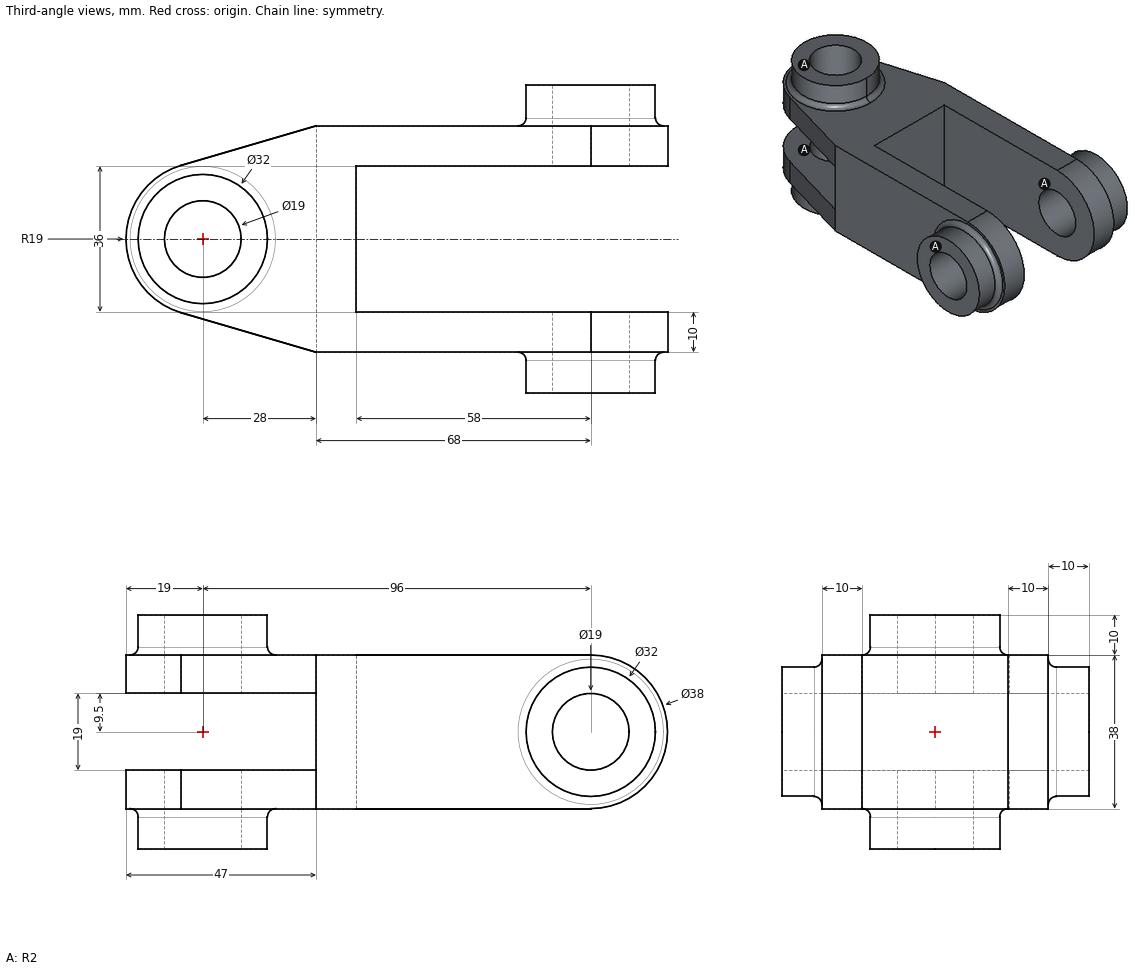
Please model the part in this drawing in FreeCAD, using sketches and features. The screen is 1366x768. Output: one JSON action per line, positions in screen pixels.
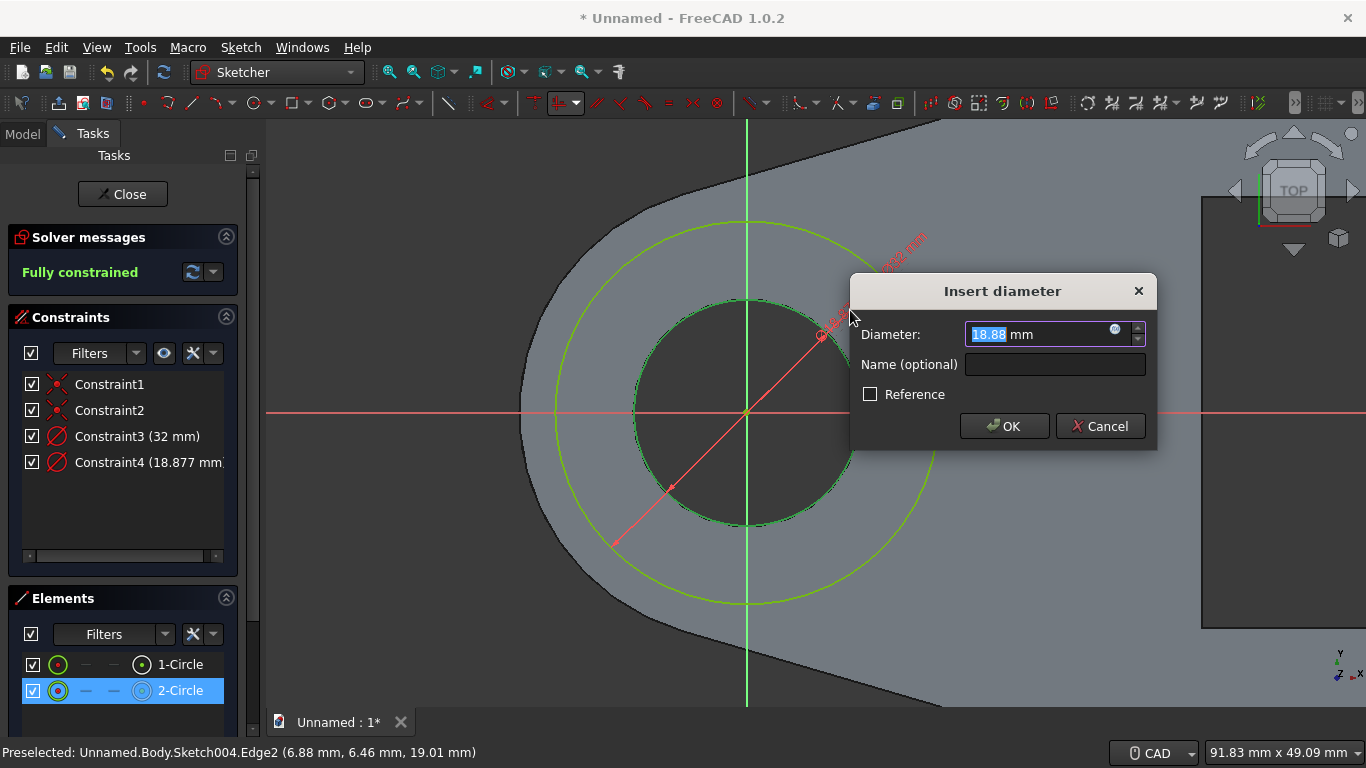
{"action": "type", "text": "19"}
{"action": "key", "text": "Return"}
{"action": "key", "text": "Escape"}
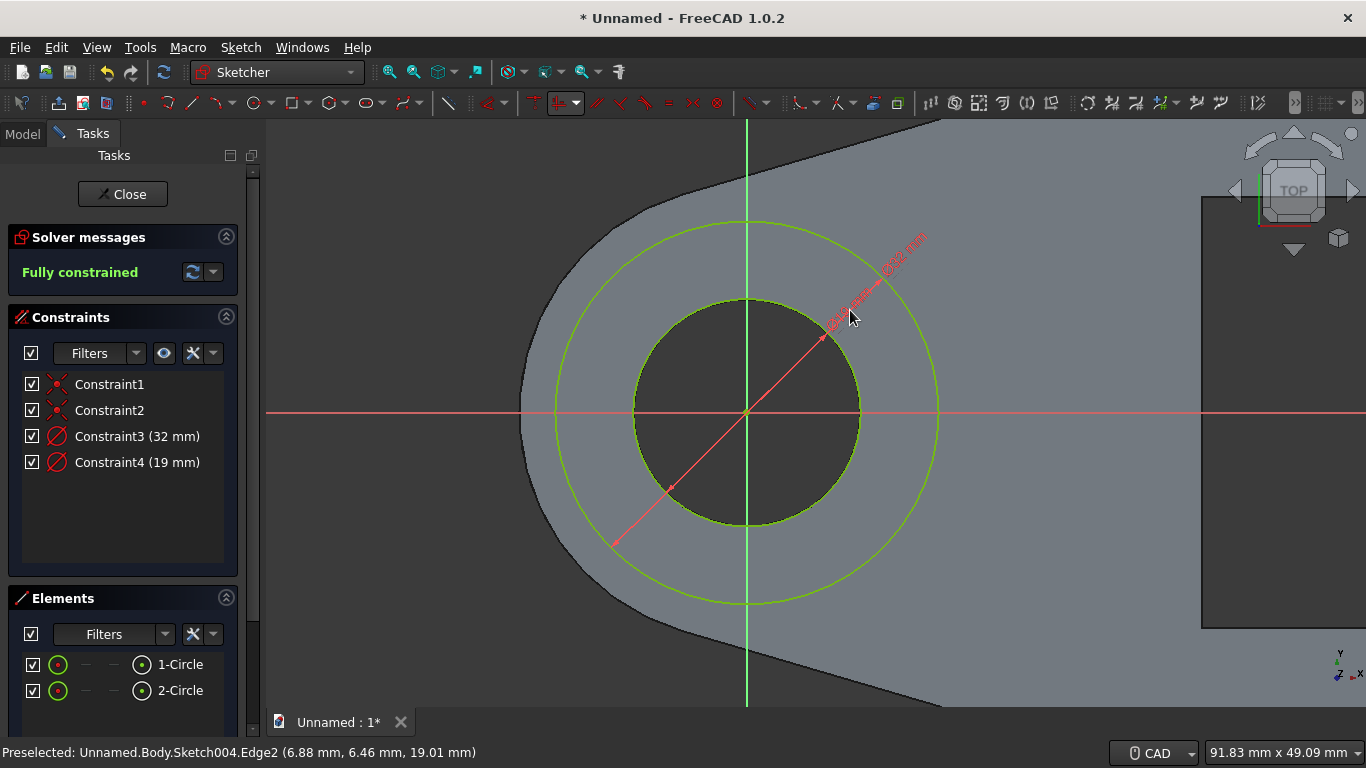
{"action": "left_click", "coordinate": [123, 194]}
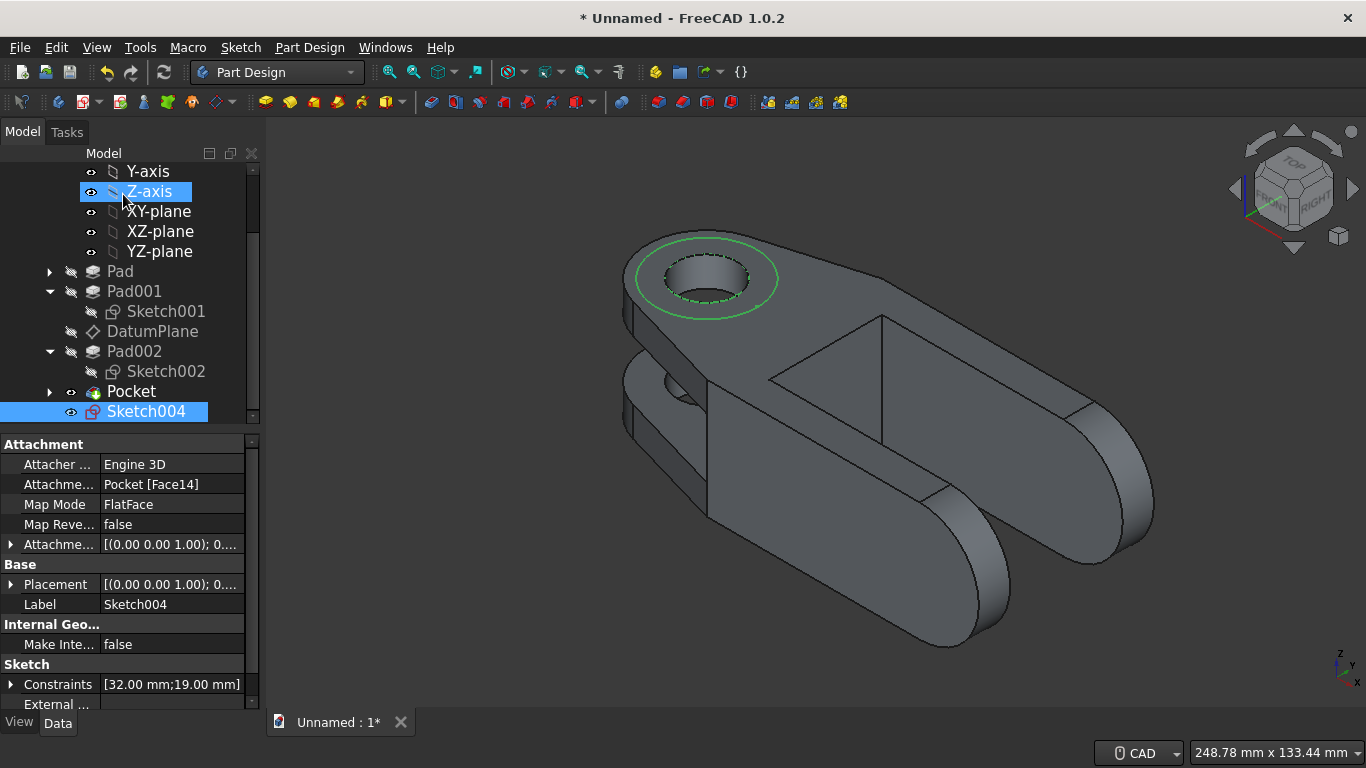
{"action": "left_click", "coordinate": [266, 102]}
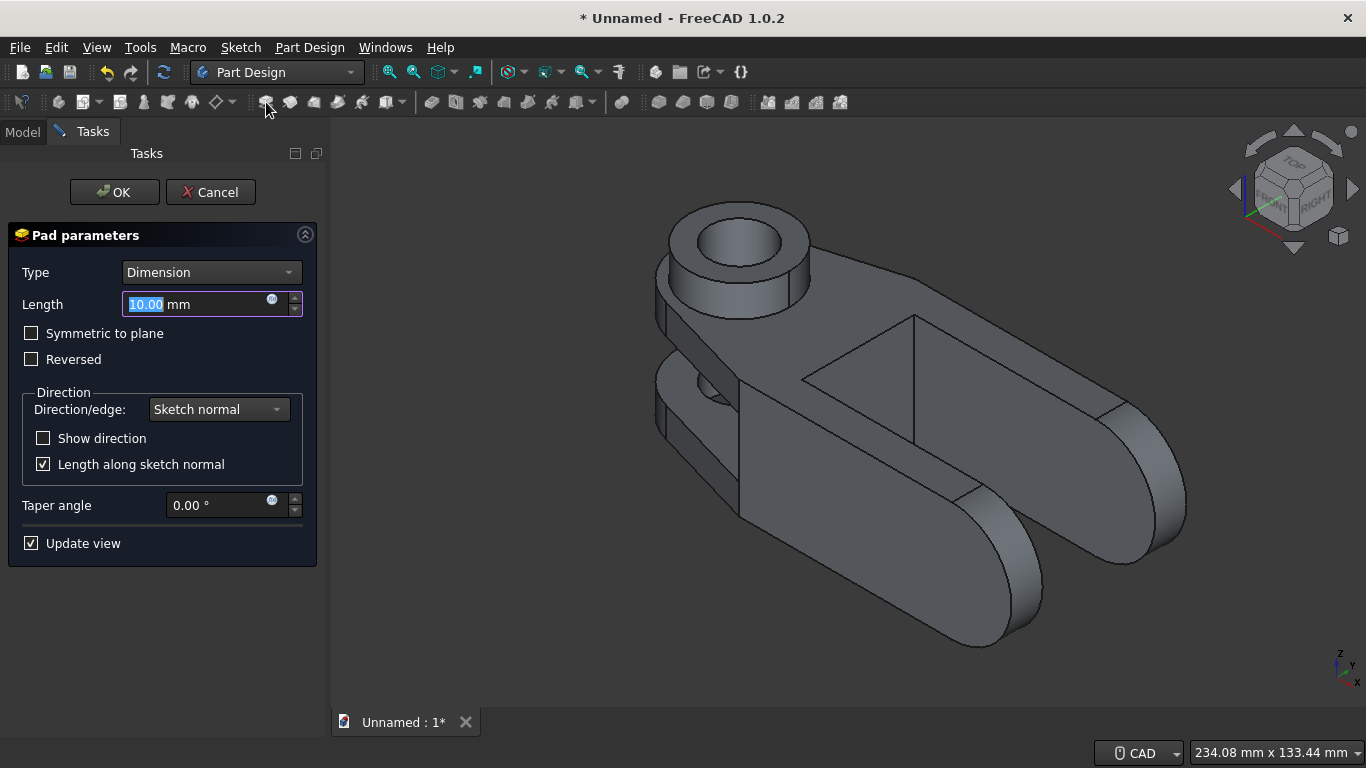
{"action": "type", "text": "10"}
{"action": "key", "text": "Tab"}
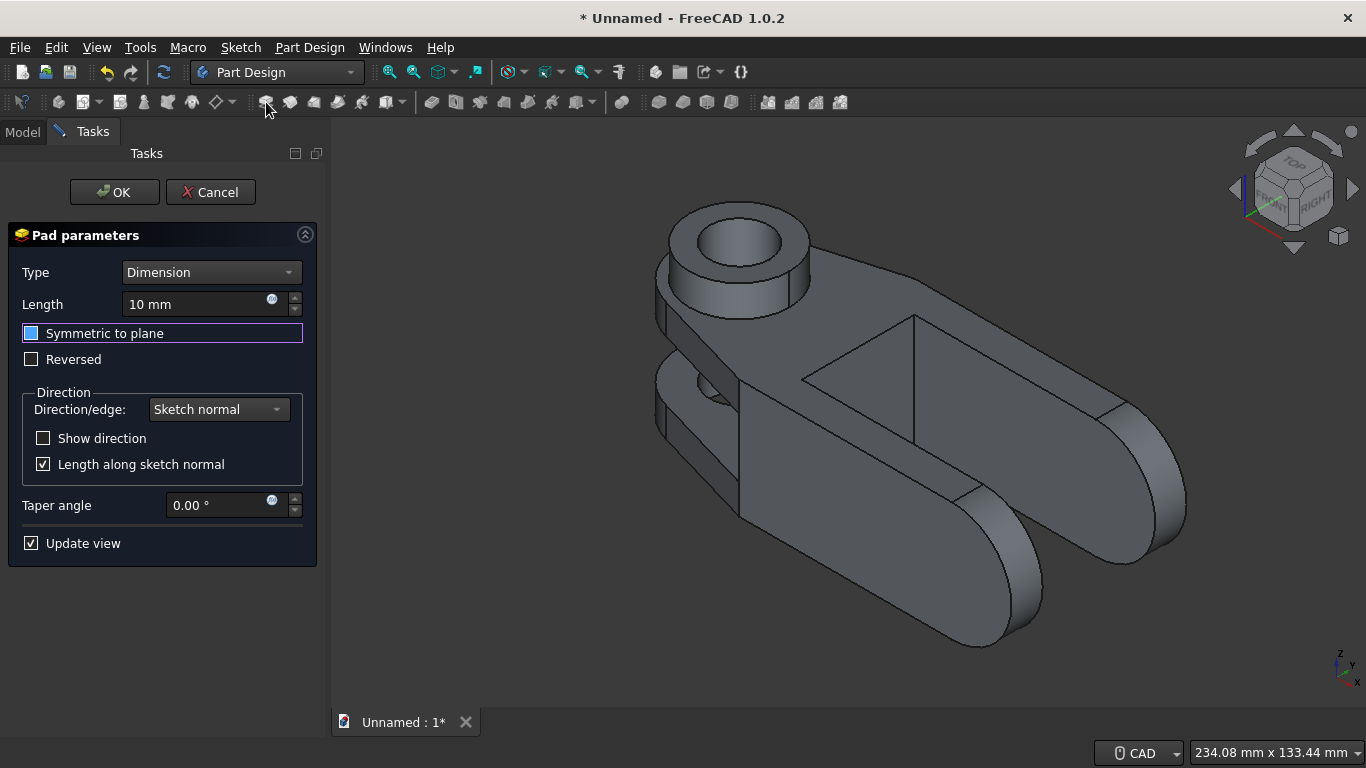
{"action": "left_click", "coordinate": [115, 192]}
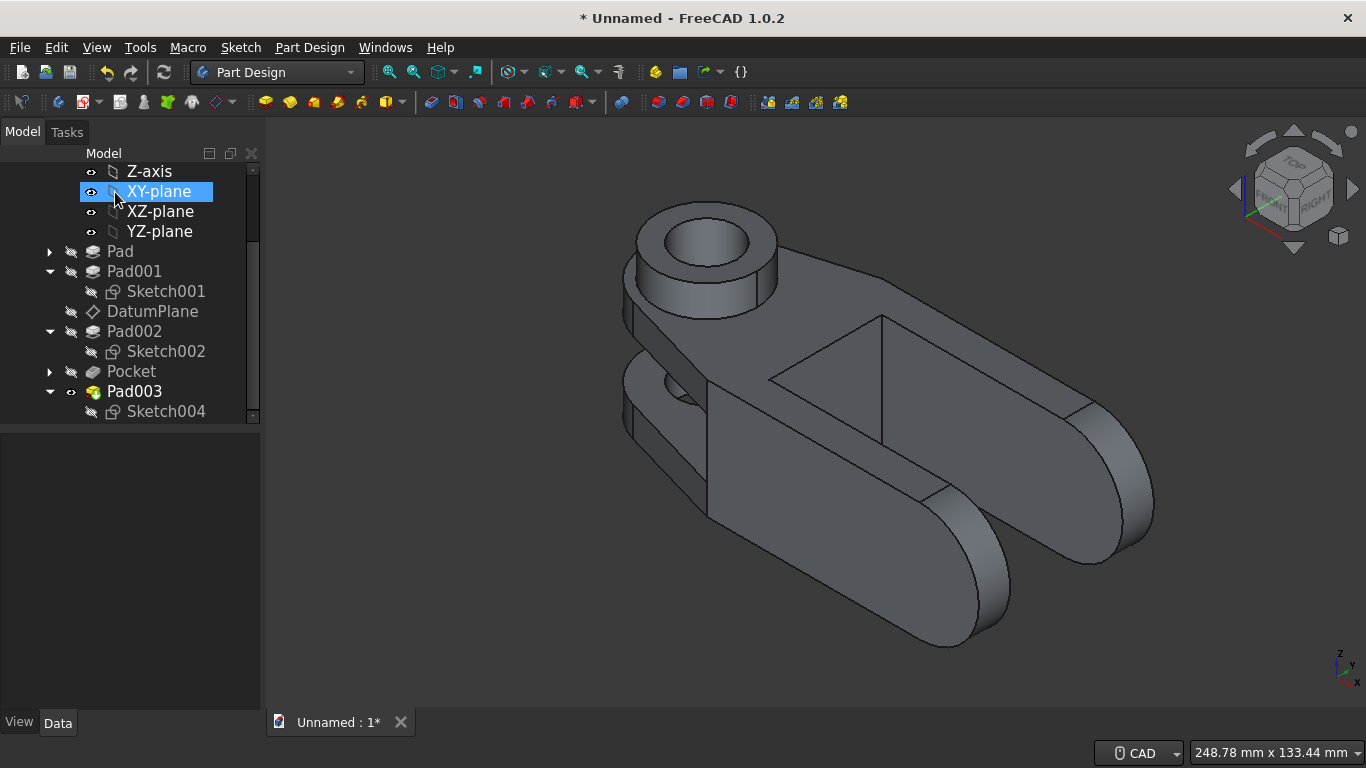
{"action": "left_click", "coordinate": [116, 392]}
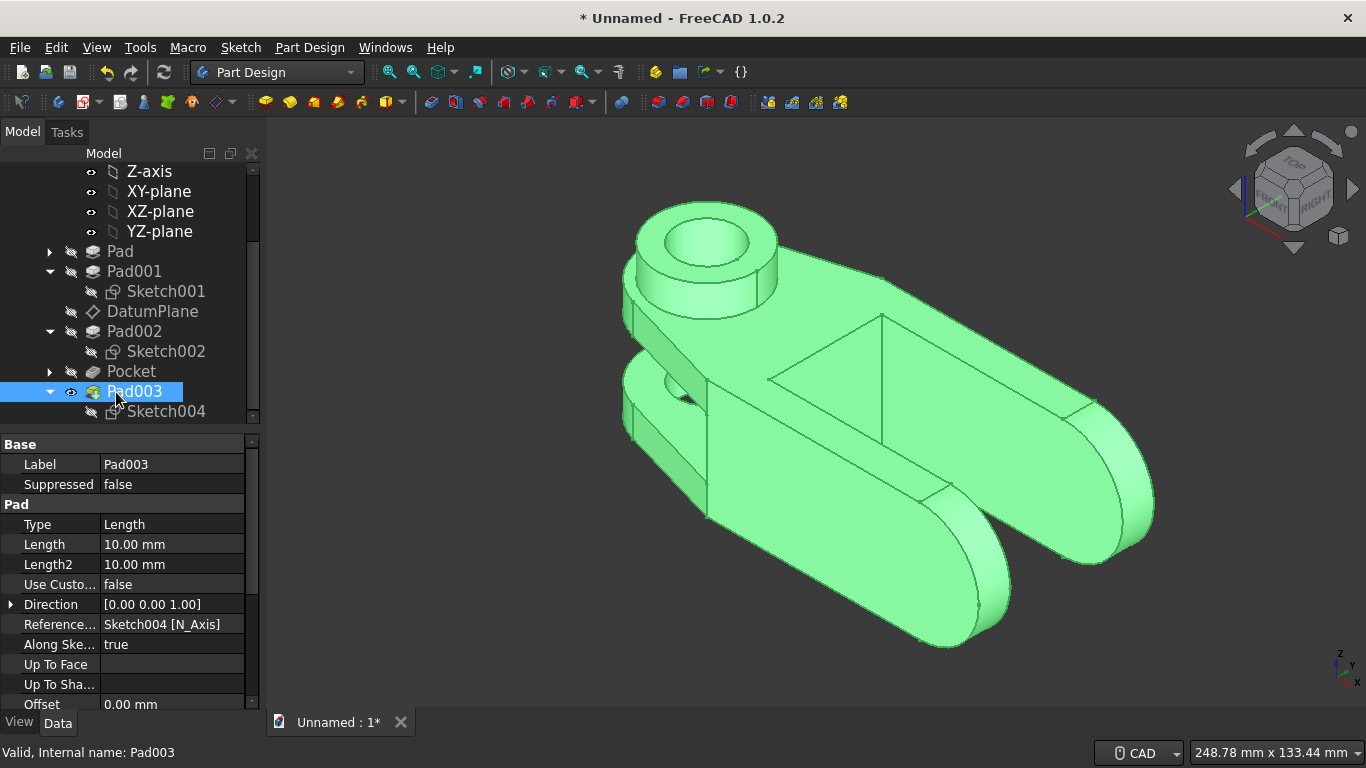
{"action": "left_click", "coordinate": [768, 102]}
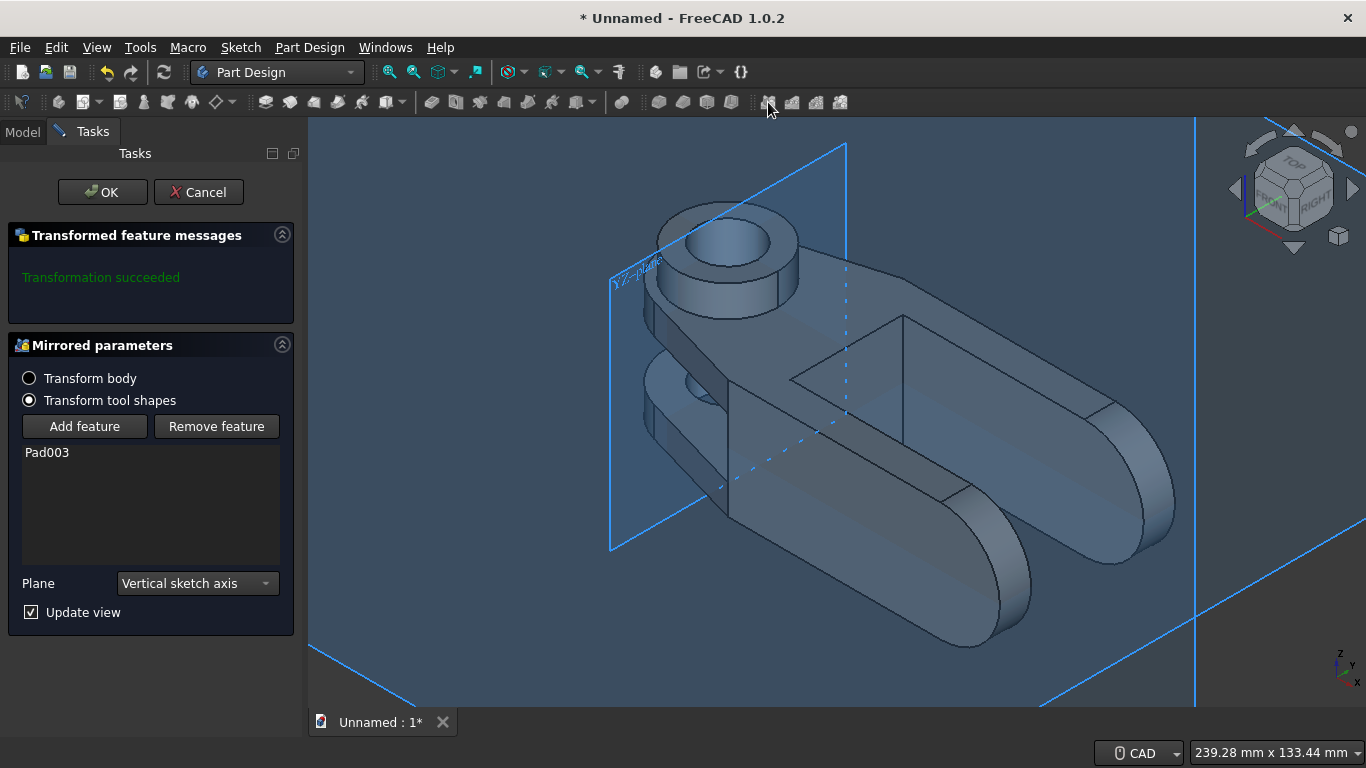
{"action": "left_click", "coordinate": [198, 584]}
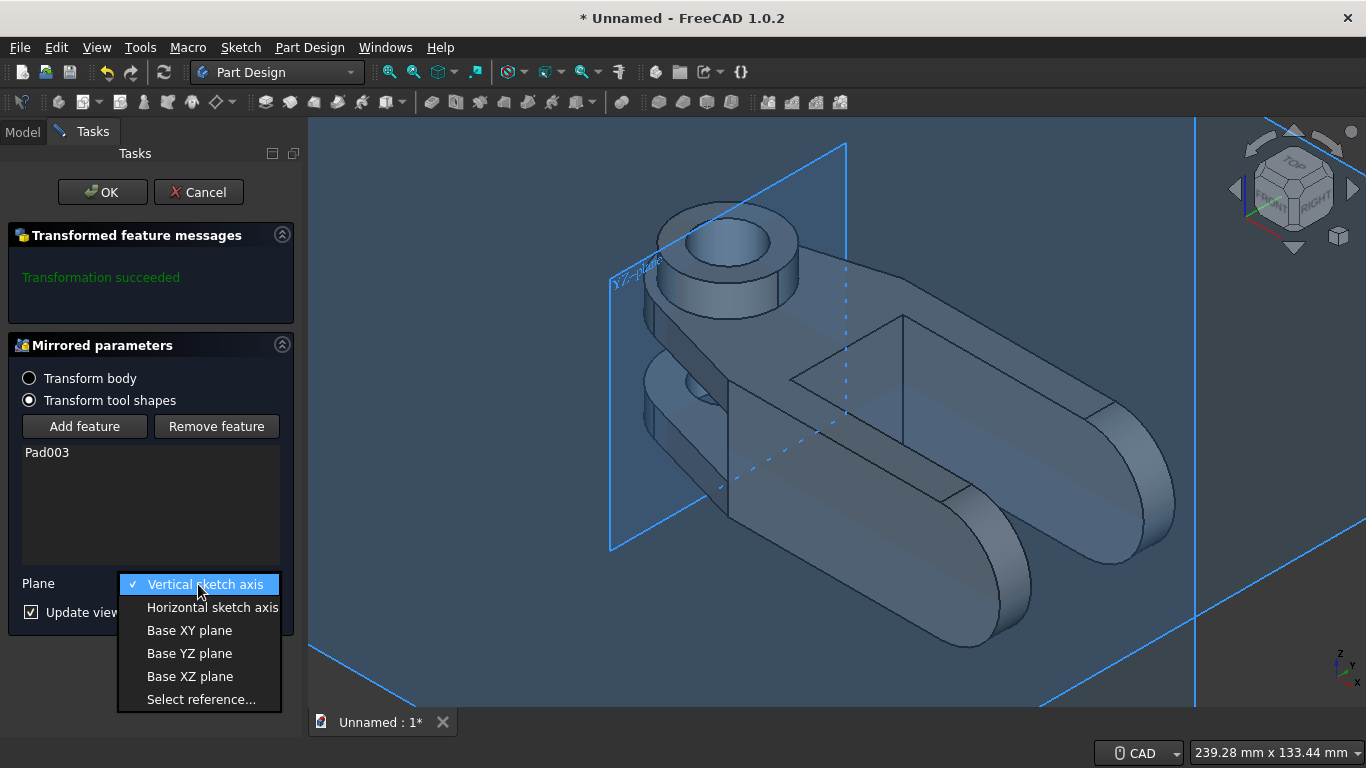
{"action": "left_click", "coordinate": [198, 630]}